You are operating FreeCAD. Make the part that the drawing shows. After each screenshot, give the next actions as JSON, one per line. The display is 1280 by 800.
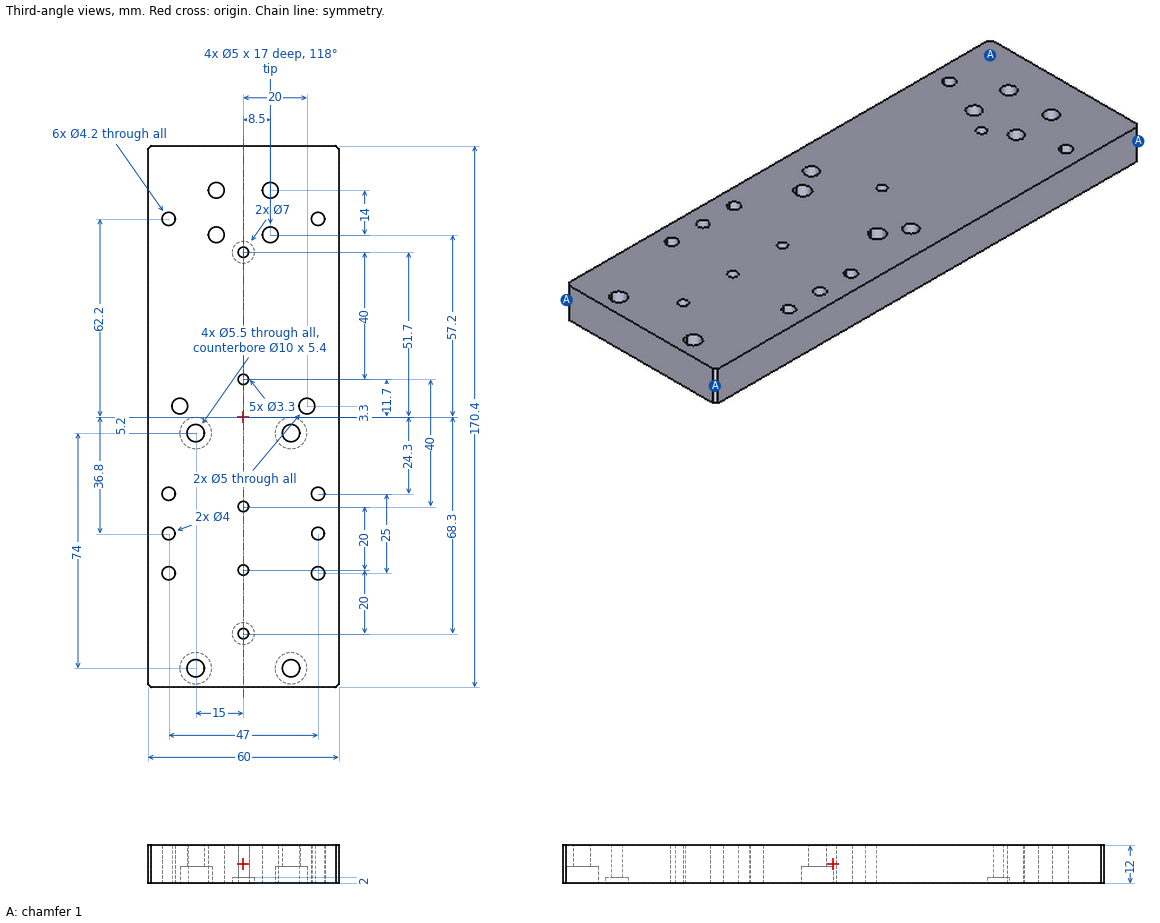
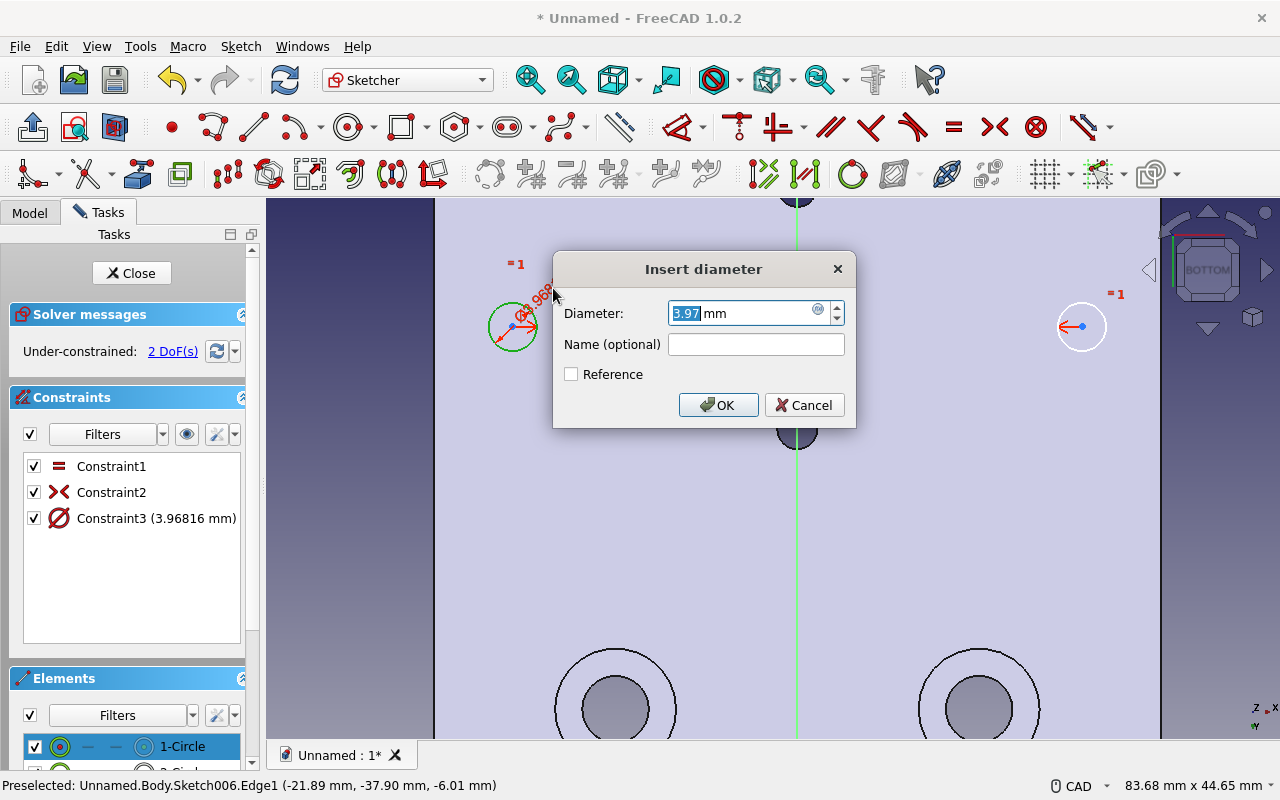
{"action": "type", "text": "4"}
{"action": "key", "text": "Return"}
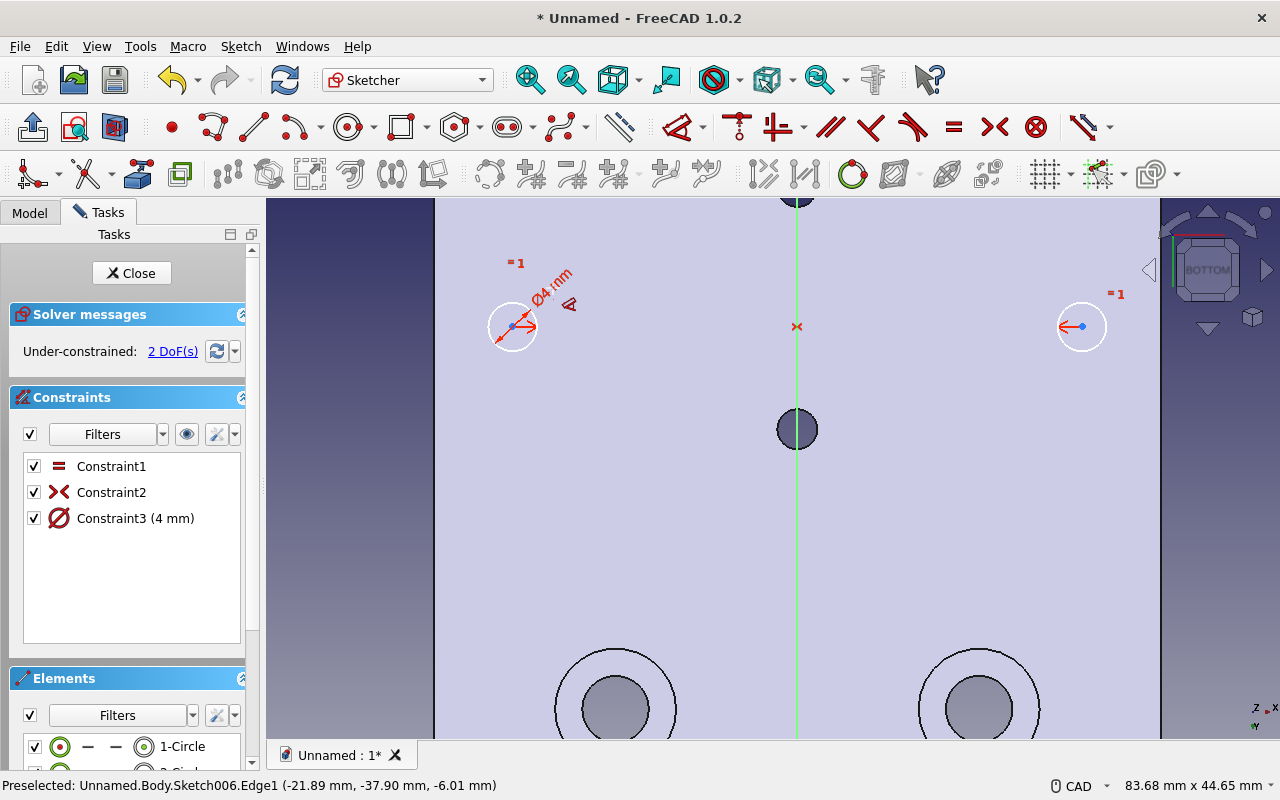
{"action": "left_click", "coordinate": [513, 327]}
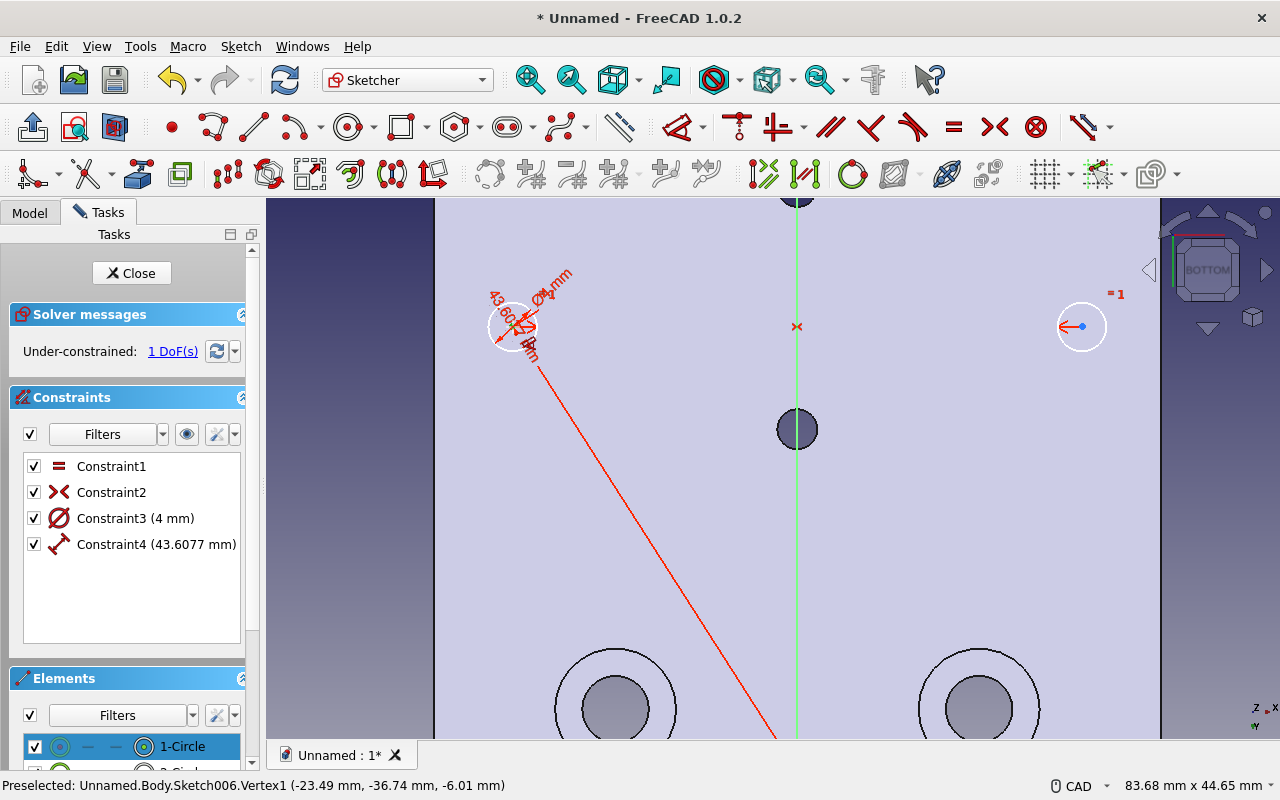
{"action": "left_click", "coordinate": [1082, 327]}
{"action": "left_click", "coordinate": [666, 293]}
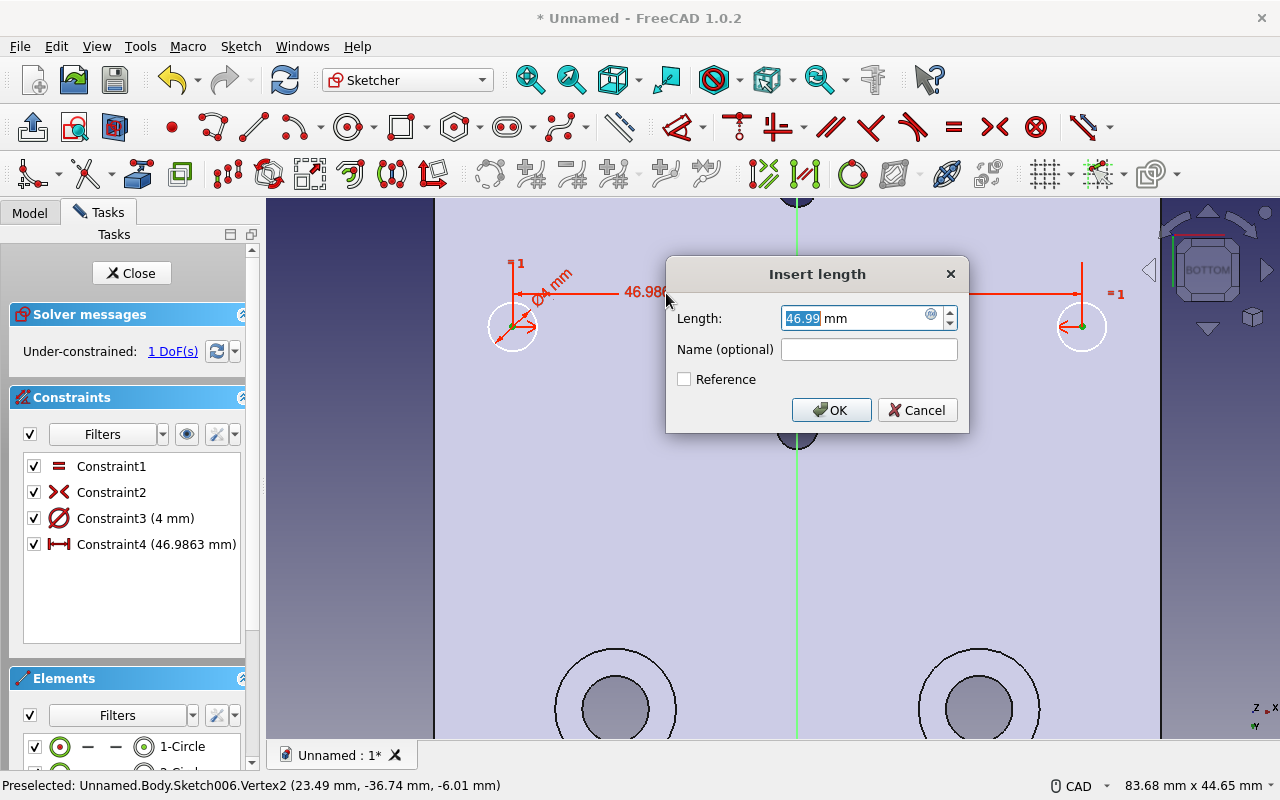
{"action": "type", "text": "47"}
{"action": "key", "text": "Return"}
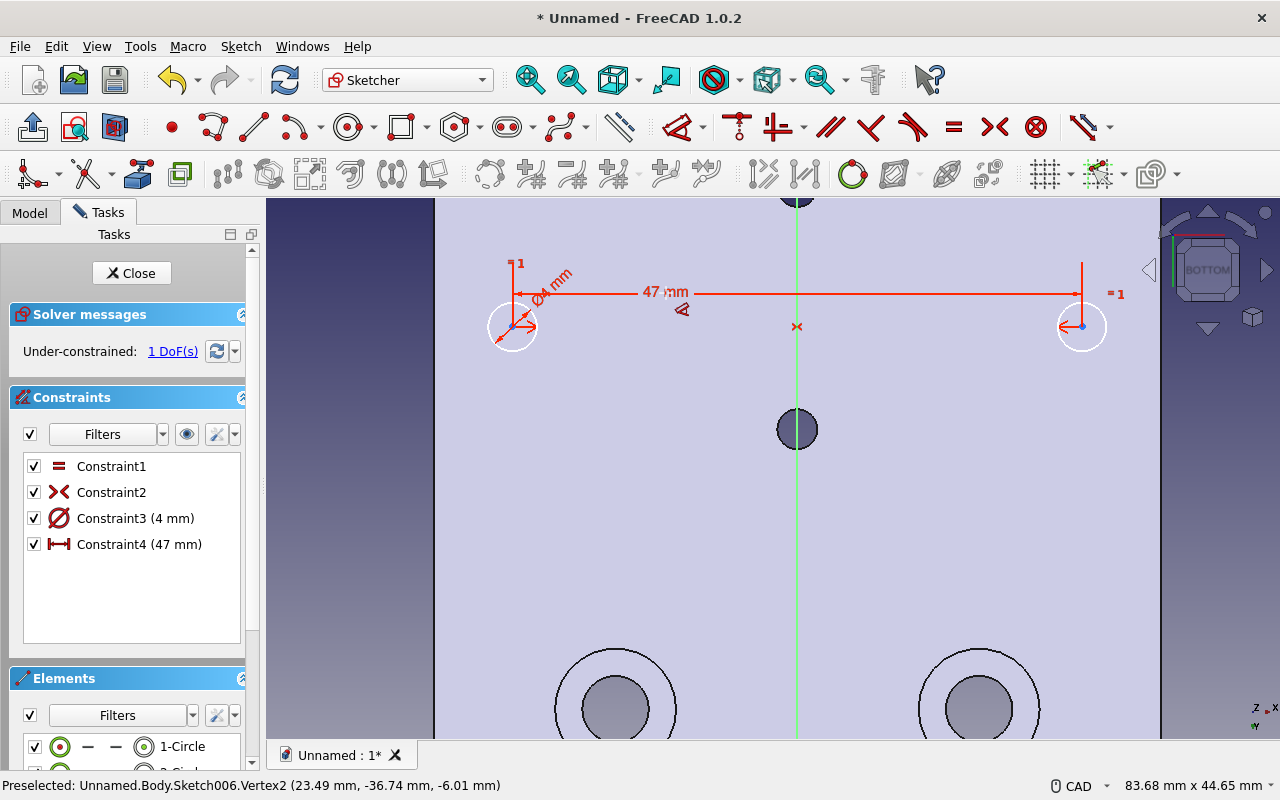
{"action": "left_click", "coordinate": [513, 327]}
{"action": "left_click", "coordinate": [479, 519]}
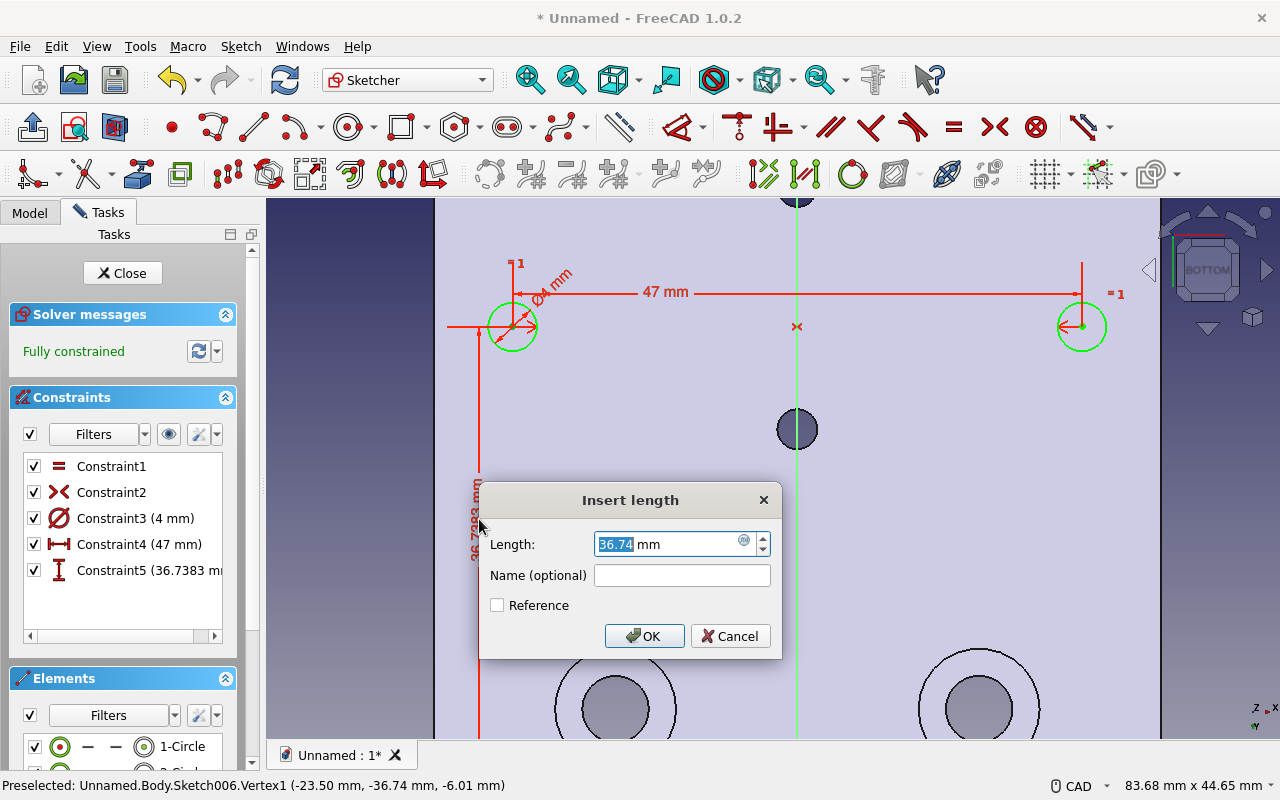
{"action": "type", "text": "36.8"}
{"action": "key", "text": "Return"}
{"action": "key", "text": "Escape"}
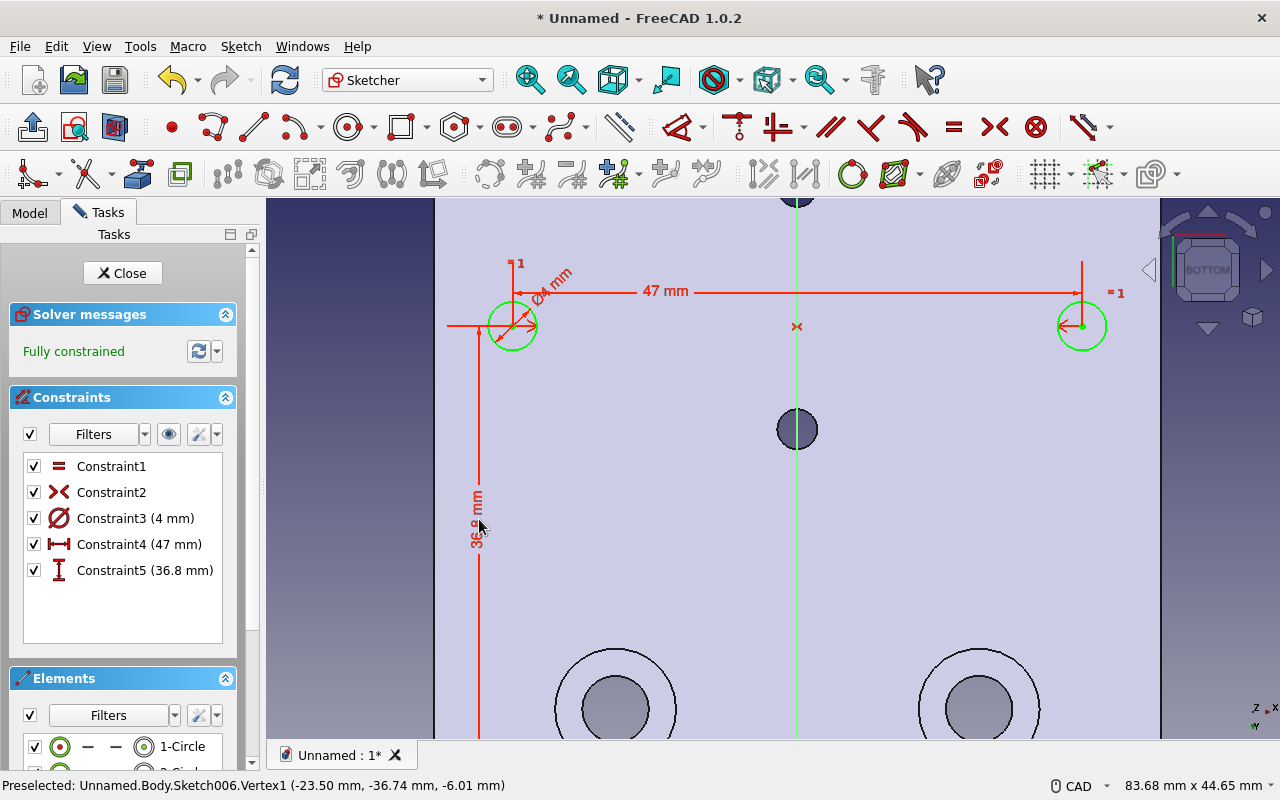
{"action": "left_click", "coordinate": [123, 273]}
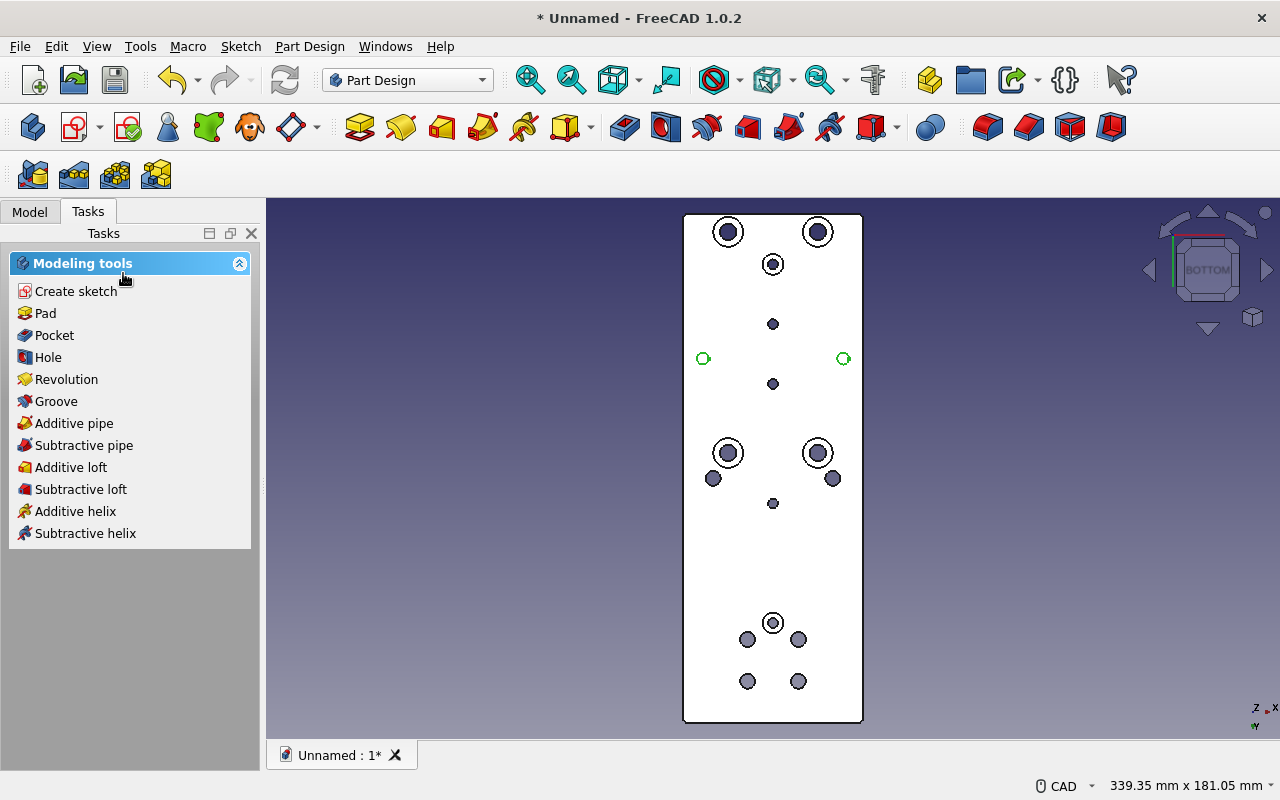
{"action": "left_click", "coordinate": [625, 128]}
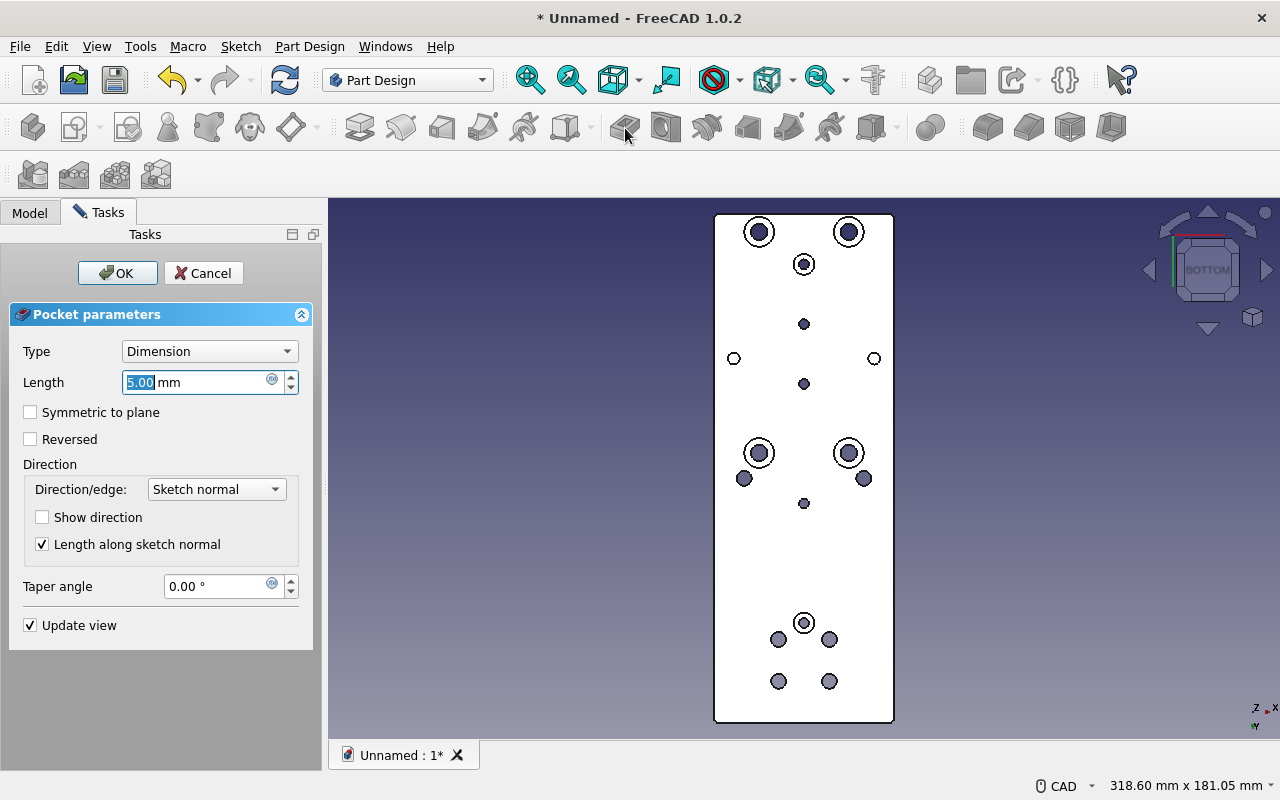
{"action": "left_click", "coordinate": [210, 352]}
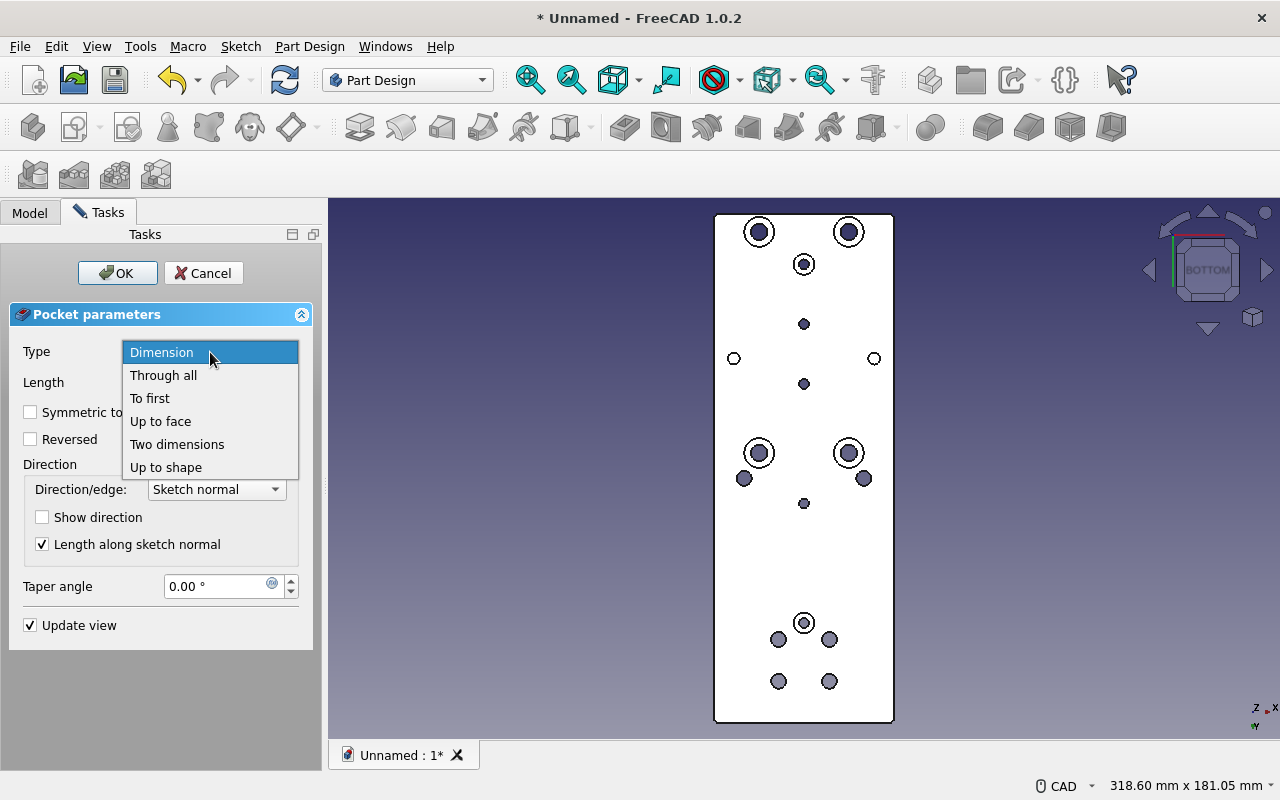
{"action": "left_click", "coordinate": [208, 376]}